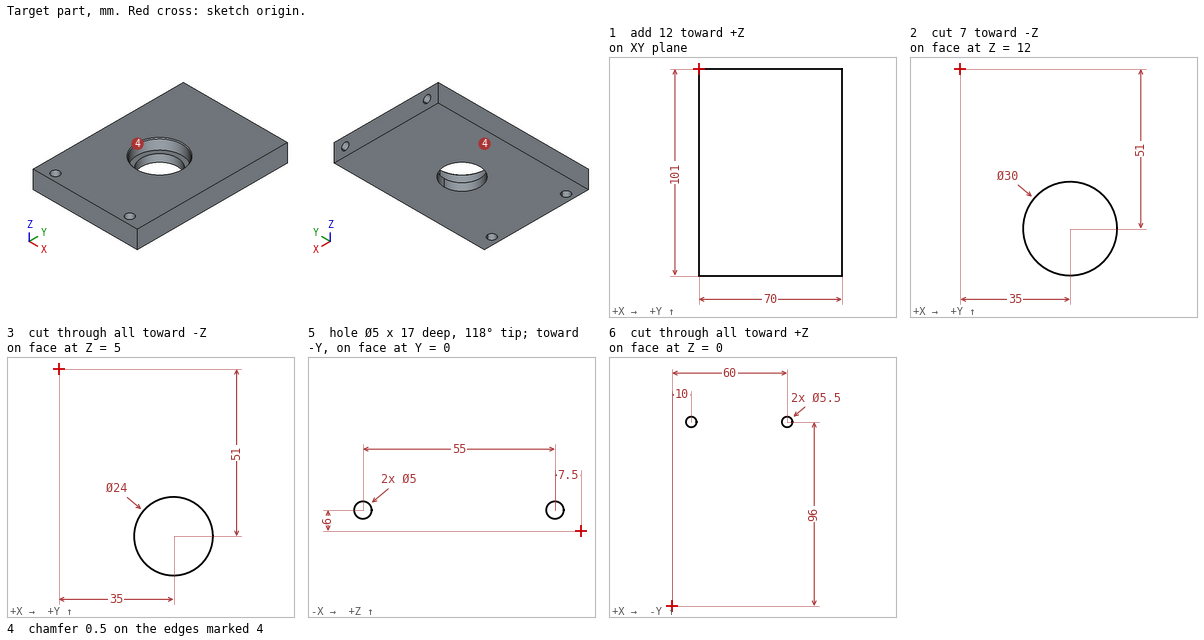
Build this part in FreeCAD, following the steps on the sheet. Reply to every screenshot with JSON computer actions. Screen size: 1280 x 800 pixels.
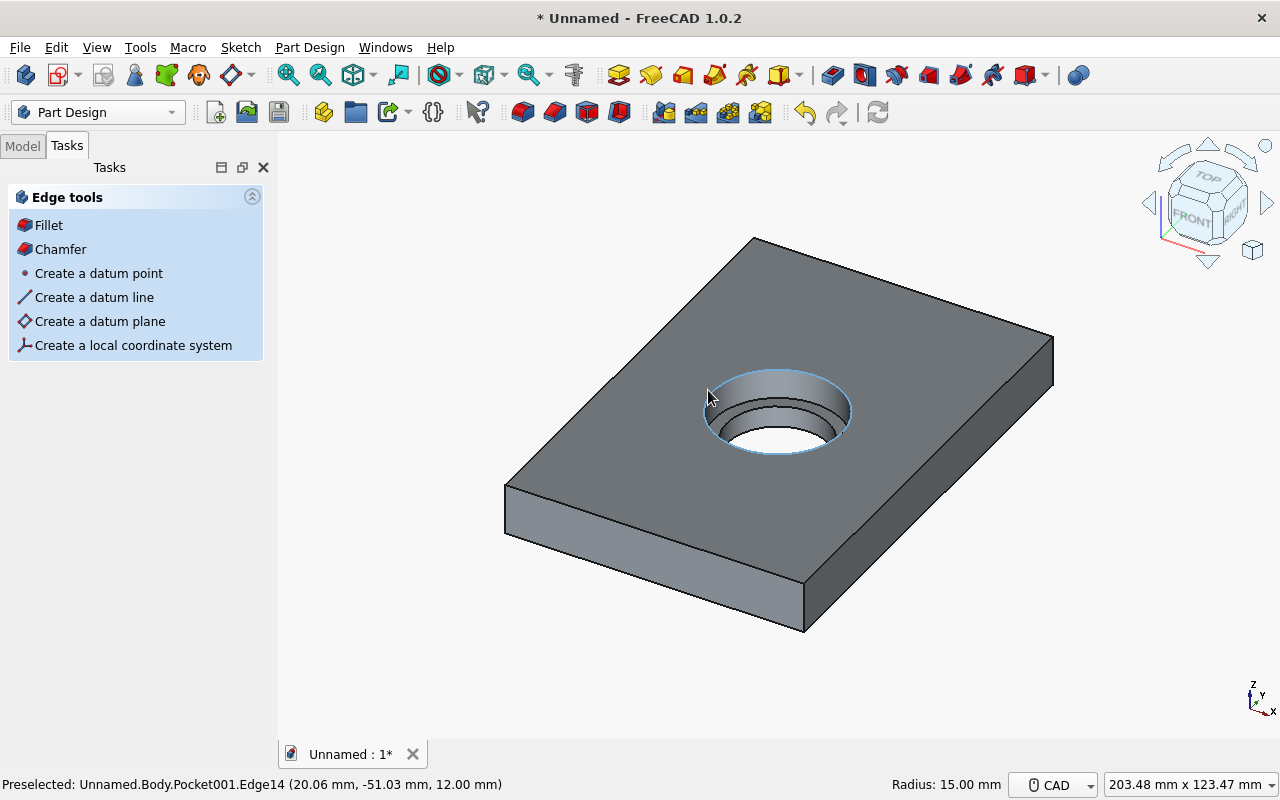
{"action": "left_click", "coordinate": [556, 112]}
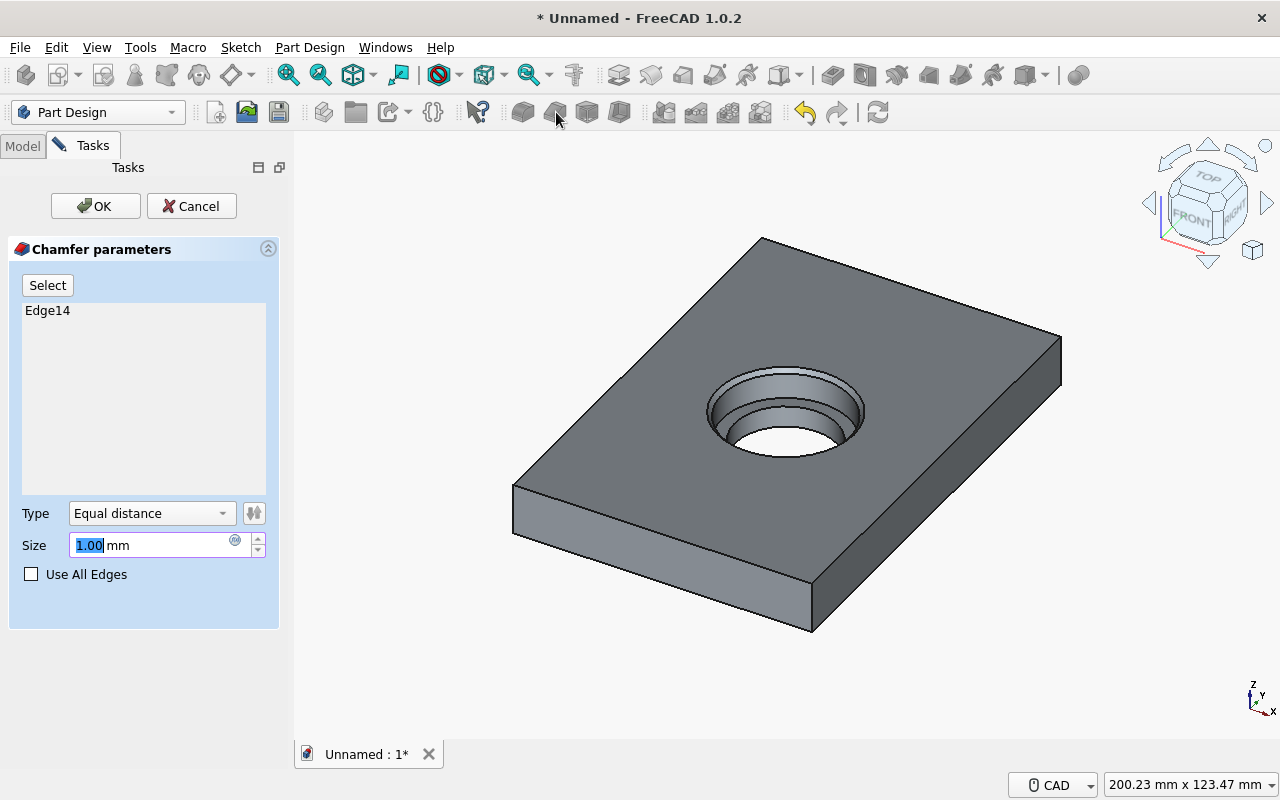
{"action": "type", "text": "0.5"}
{"action": "key", "text": "Tab"}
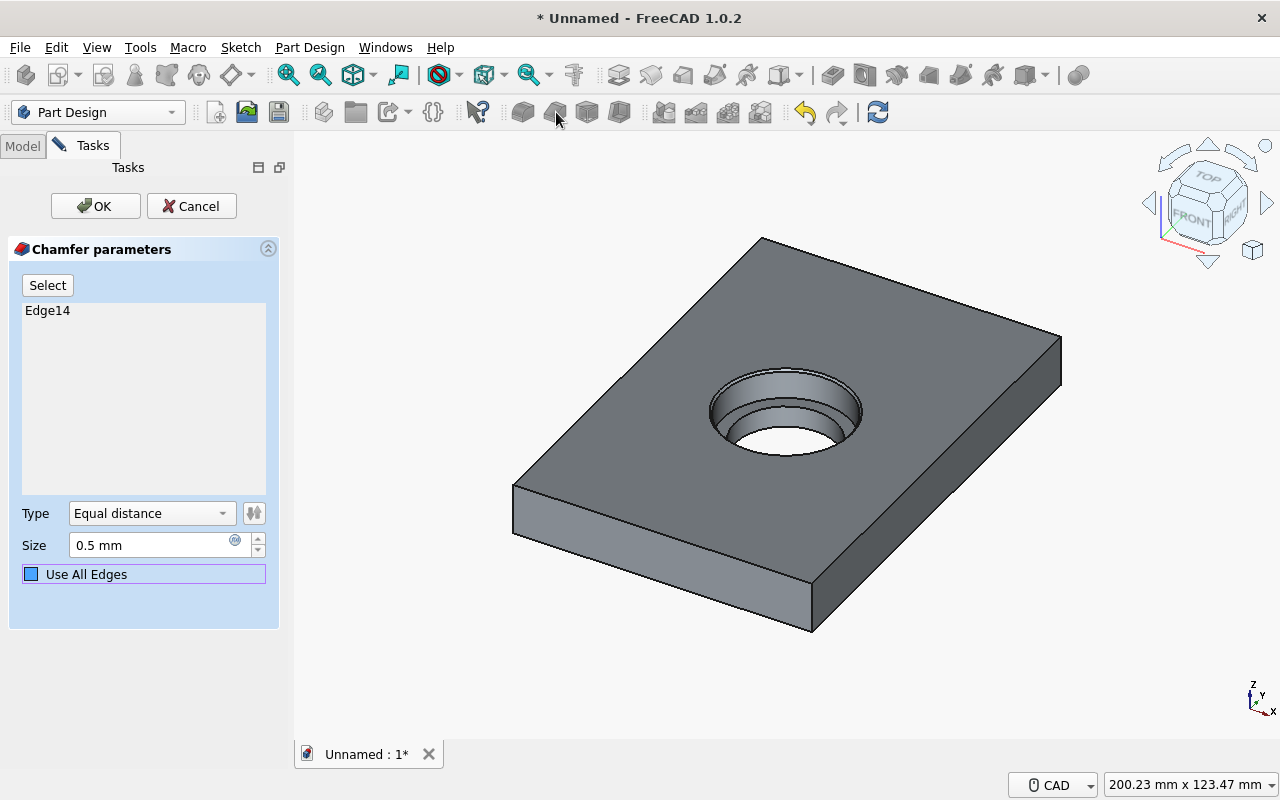
{"action": "left_click", "coordinate": [96, 206]}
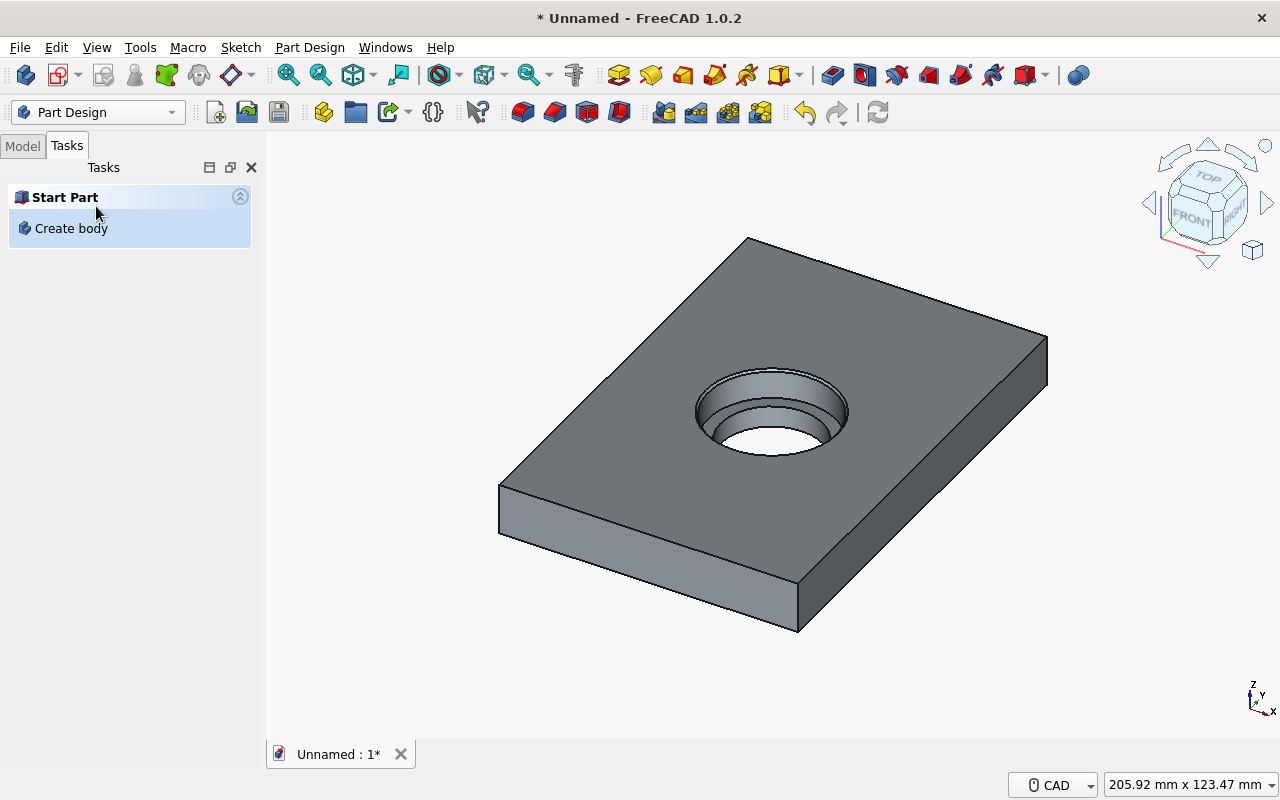
{"action": "key", "text": "4"}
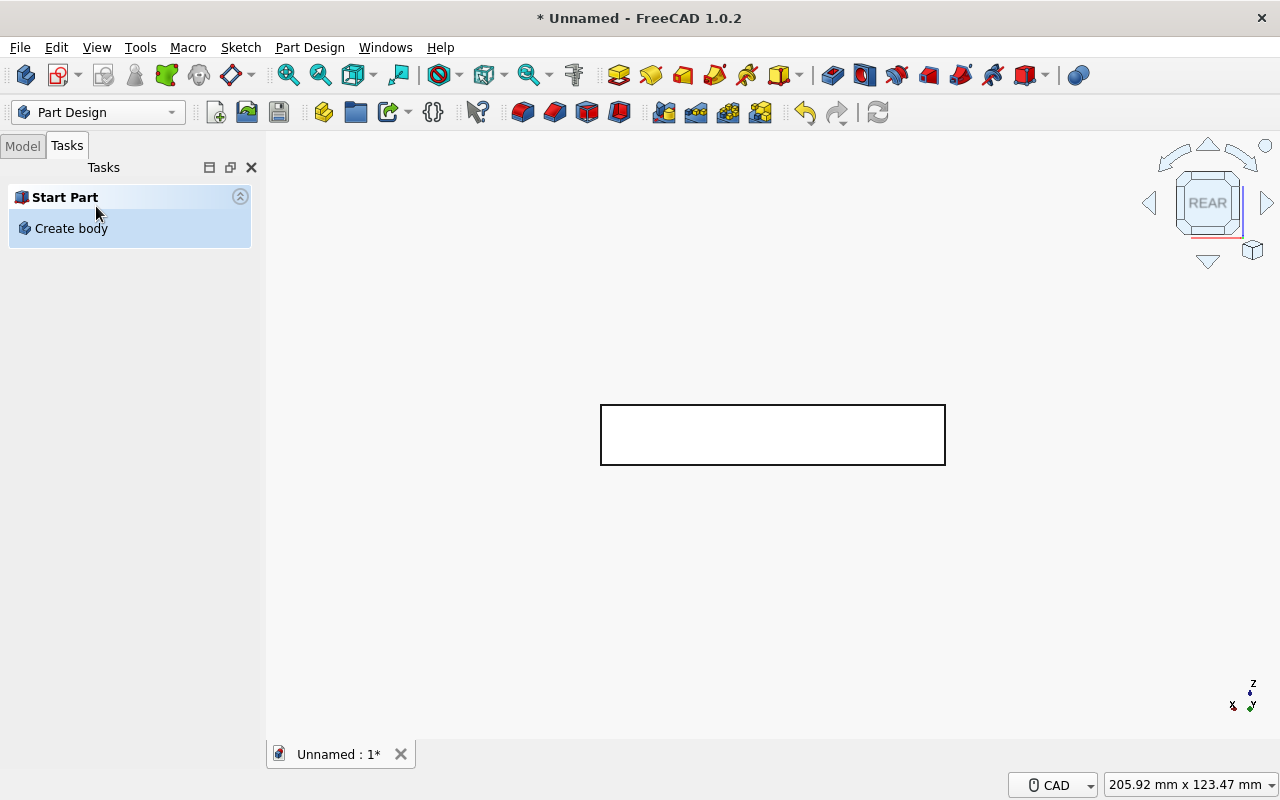
{"action": "left_click", "coordinate": [290, 76]}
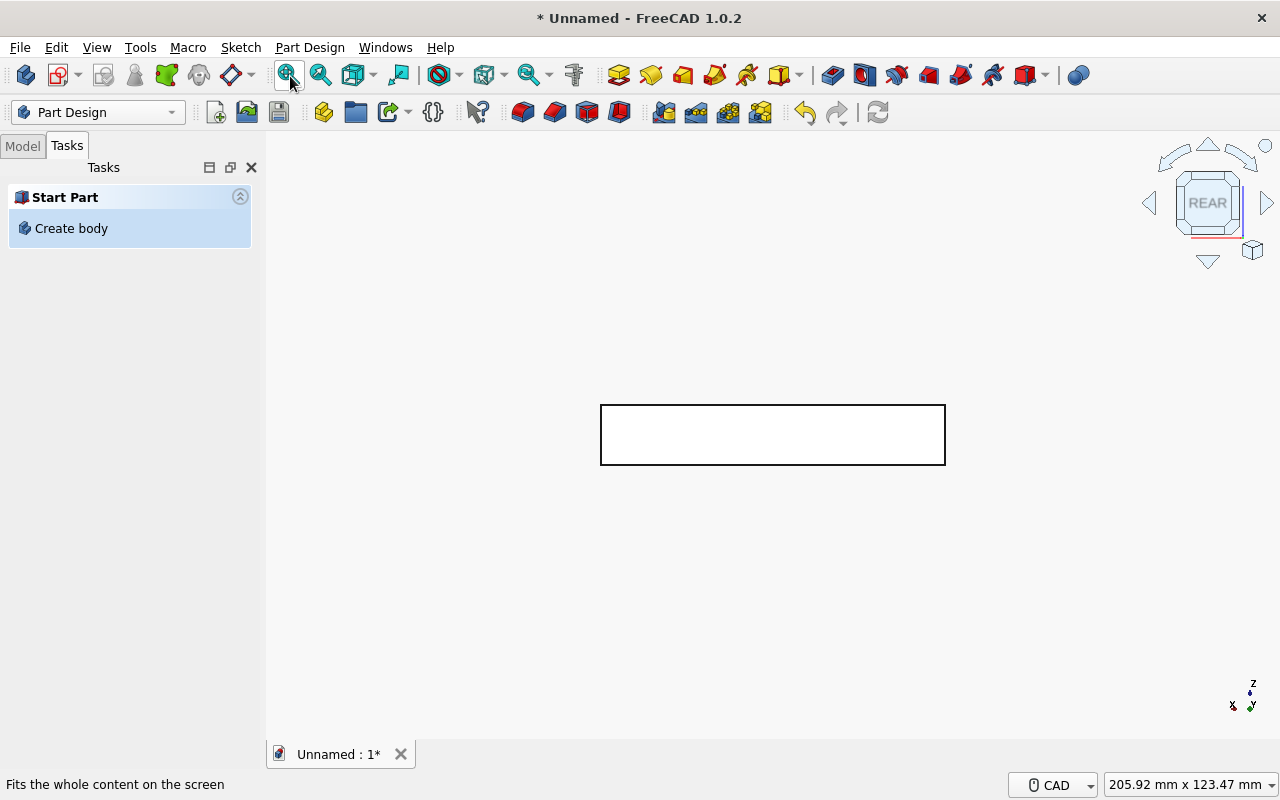
{"action": "left_click", "coordinate": [675, 434]}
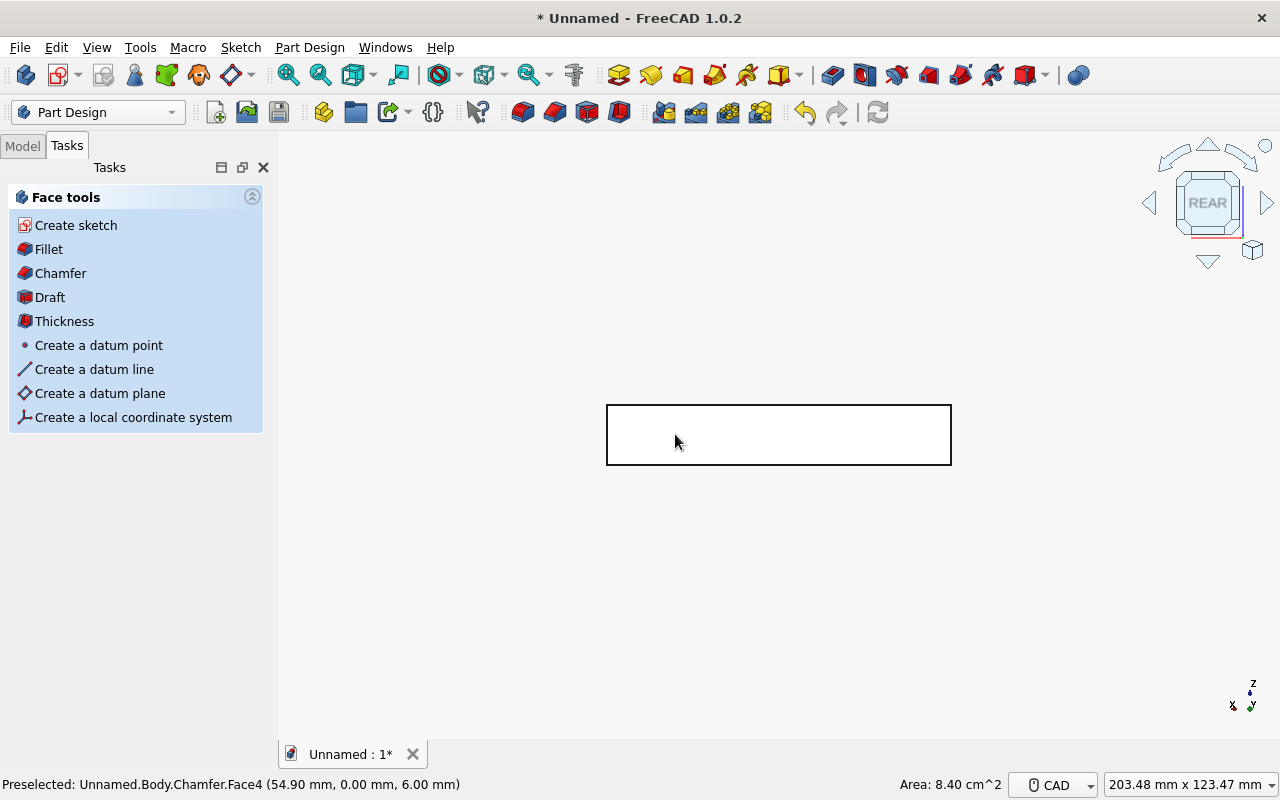
{"action": "left_click", "coordinate": [58, 76]}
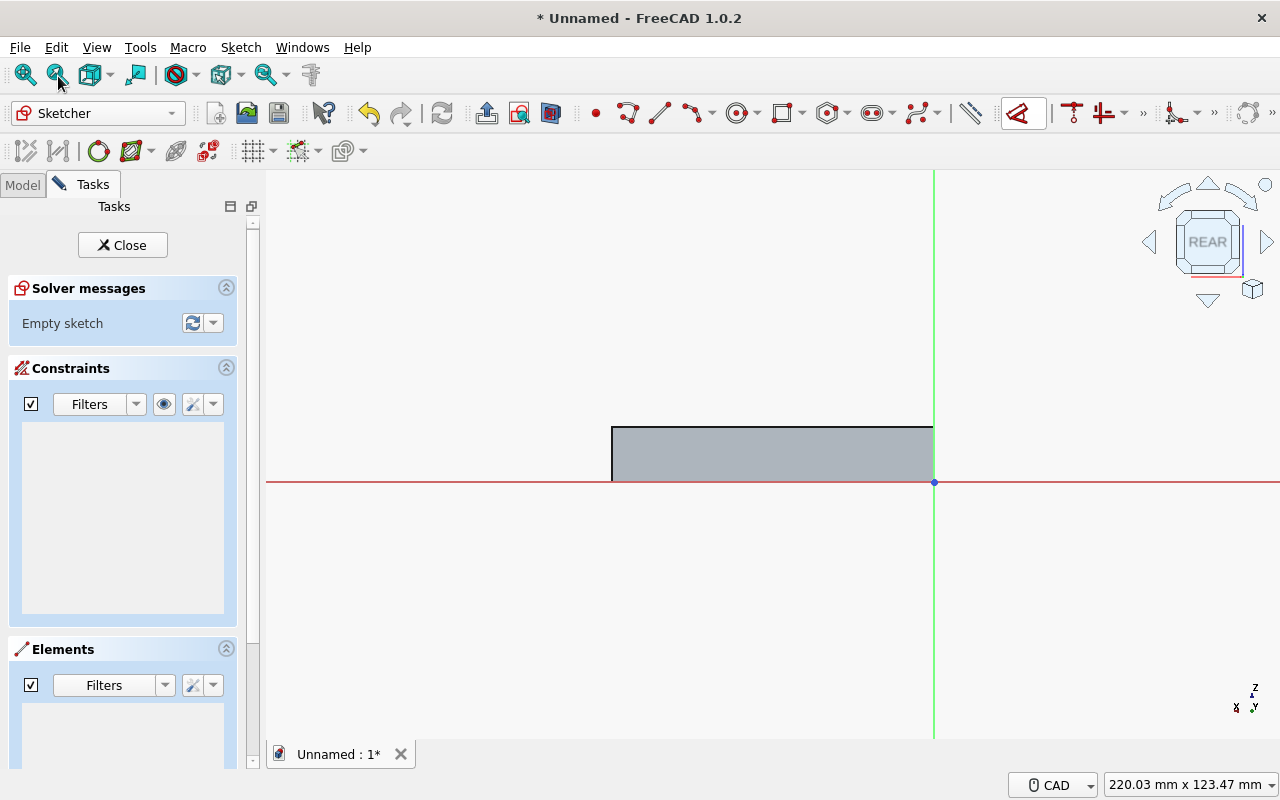
{"action": "scroll", "coordinate": [882, 472], "scroll_direction": "up", "scroll_amount": 3}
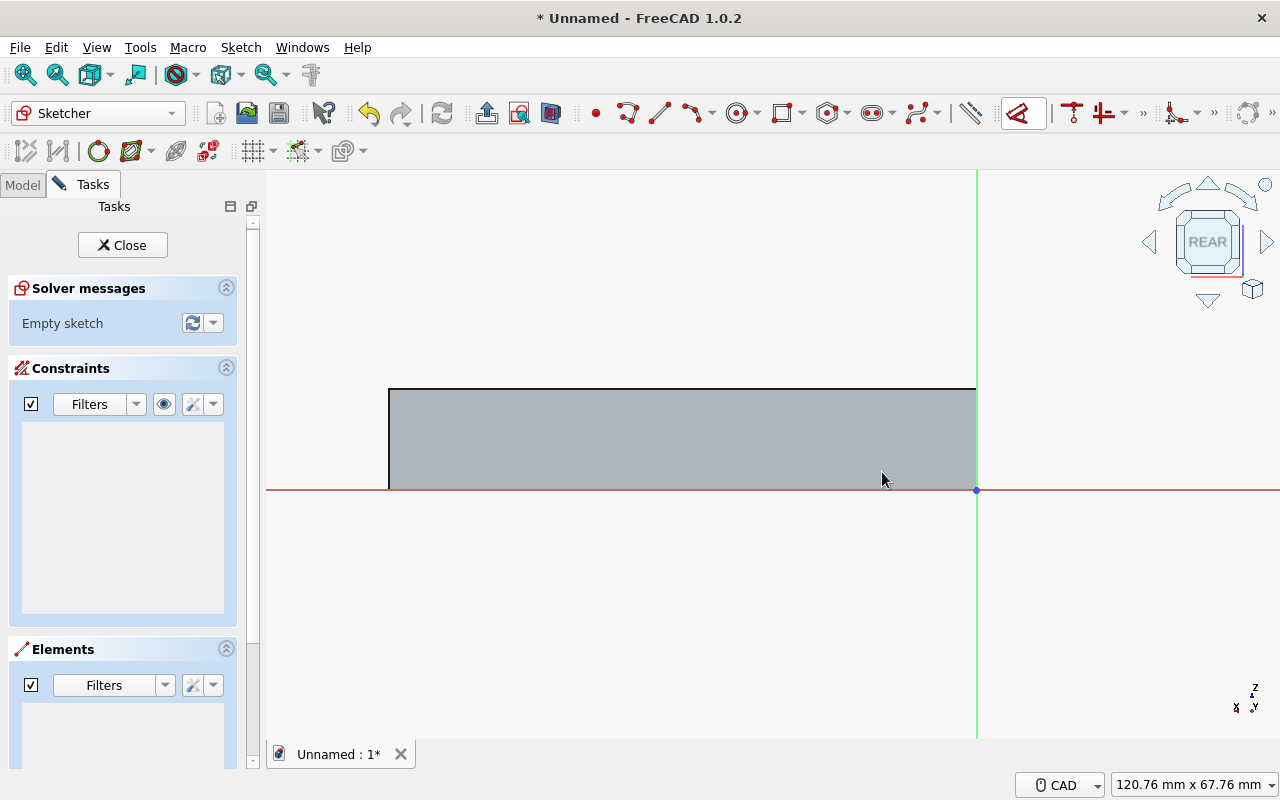
{"action": "left_click", "coordinate": [738, 114]}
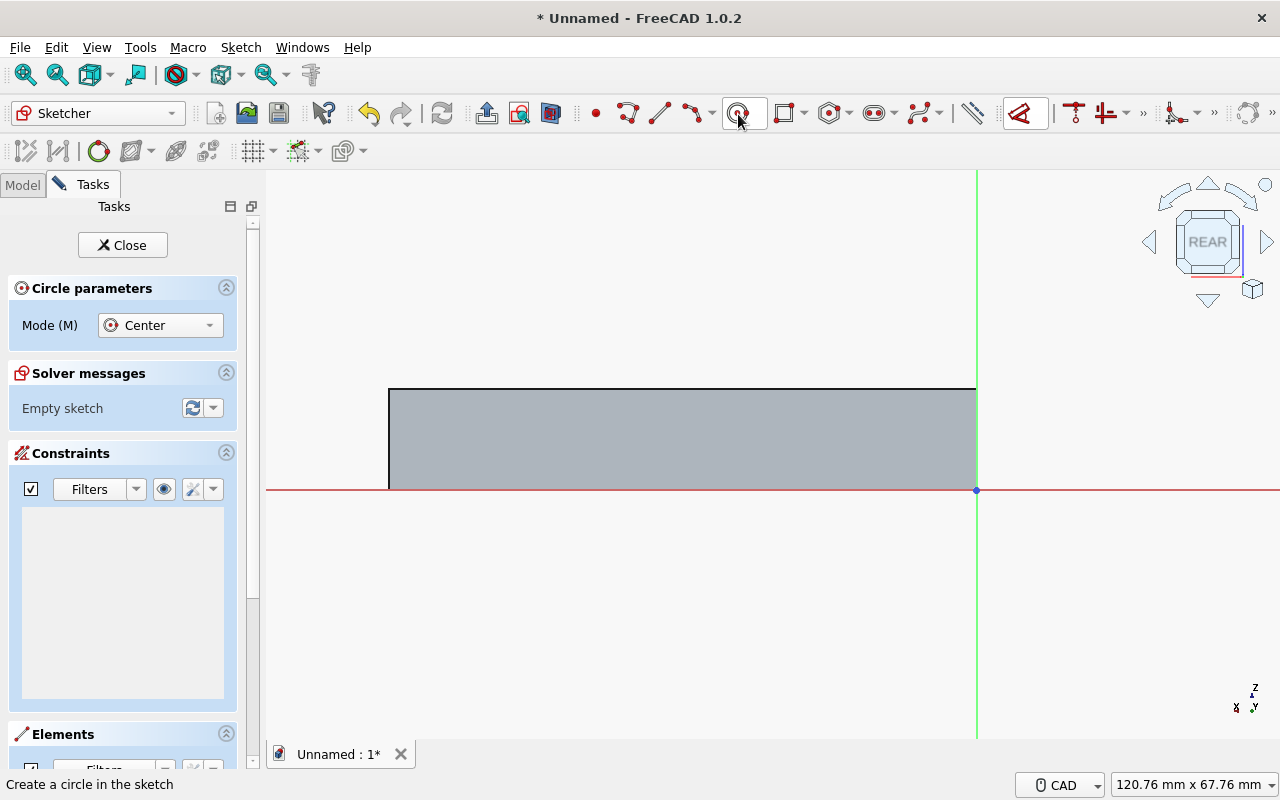
{"action": "left_click", "coordinate": [452, 440]}
{"action": "left_click", "coordinate": [467, 425]}